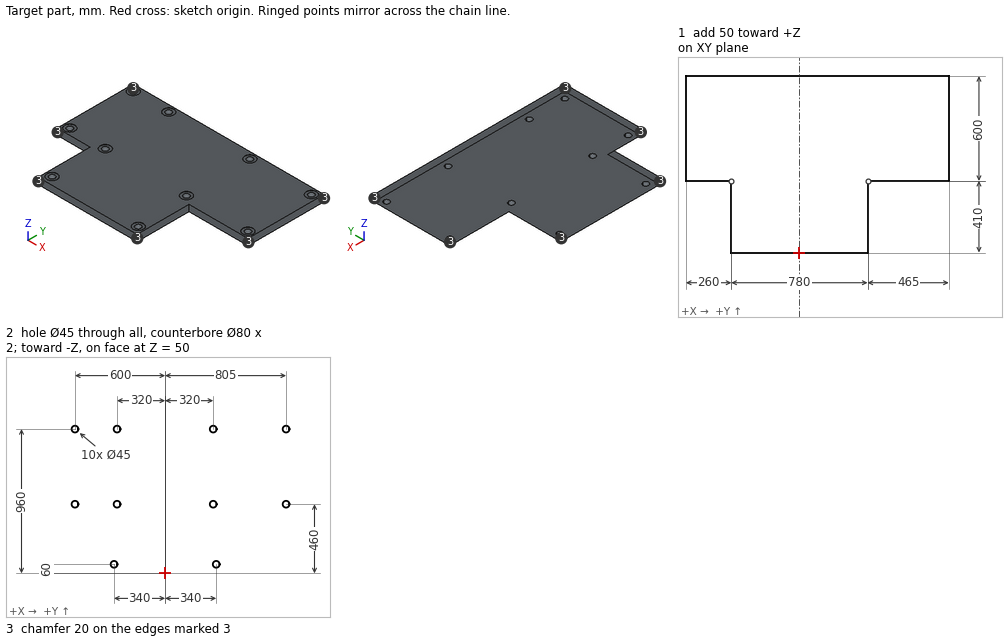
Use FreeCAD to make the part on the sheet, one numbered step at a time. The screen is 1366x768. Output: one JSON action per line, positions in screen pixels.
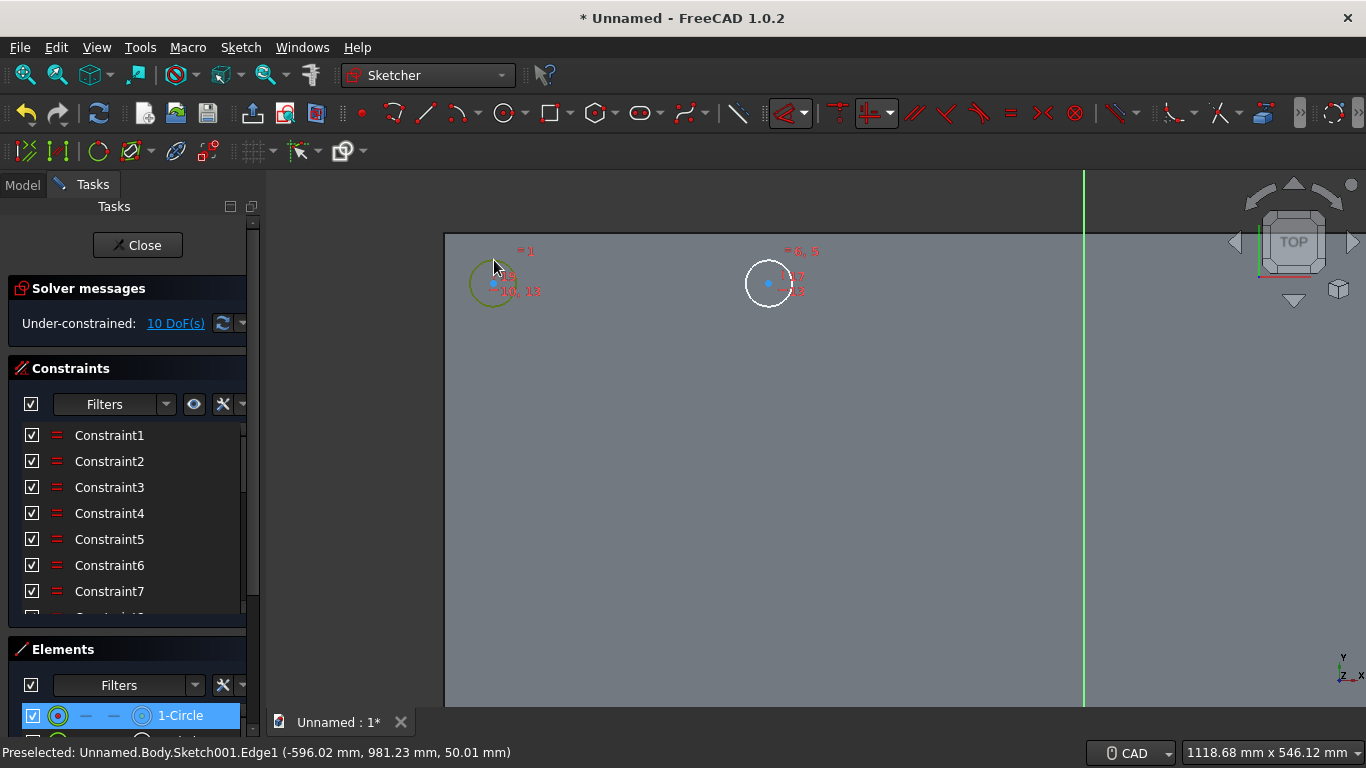
{"action": "key", "text": "k o"}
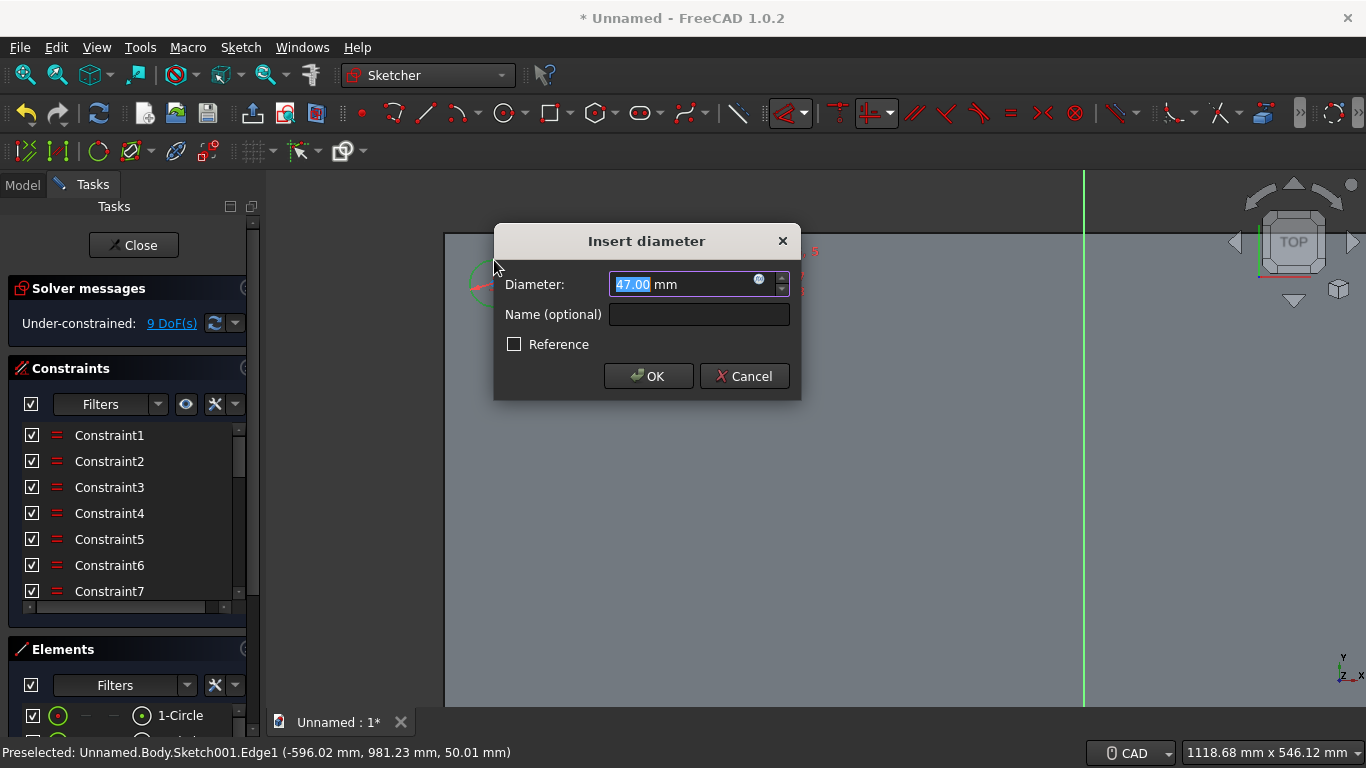
{"action": "type", "text": "45"}
{"action": "key", "text": "Return"}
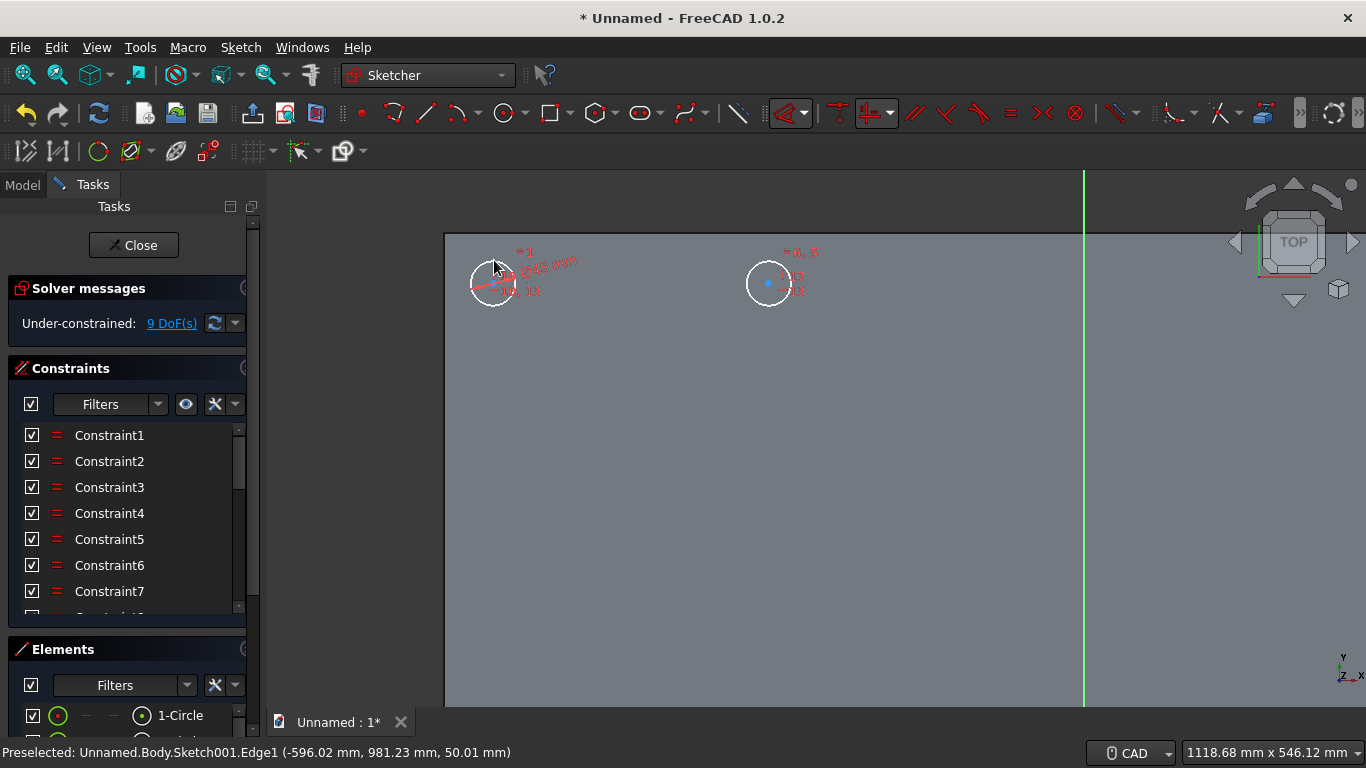
{"action": "scroll", "coordinate": [493, 262], "scroll_direction": "down", "scroll_amount": 5}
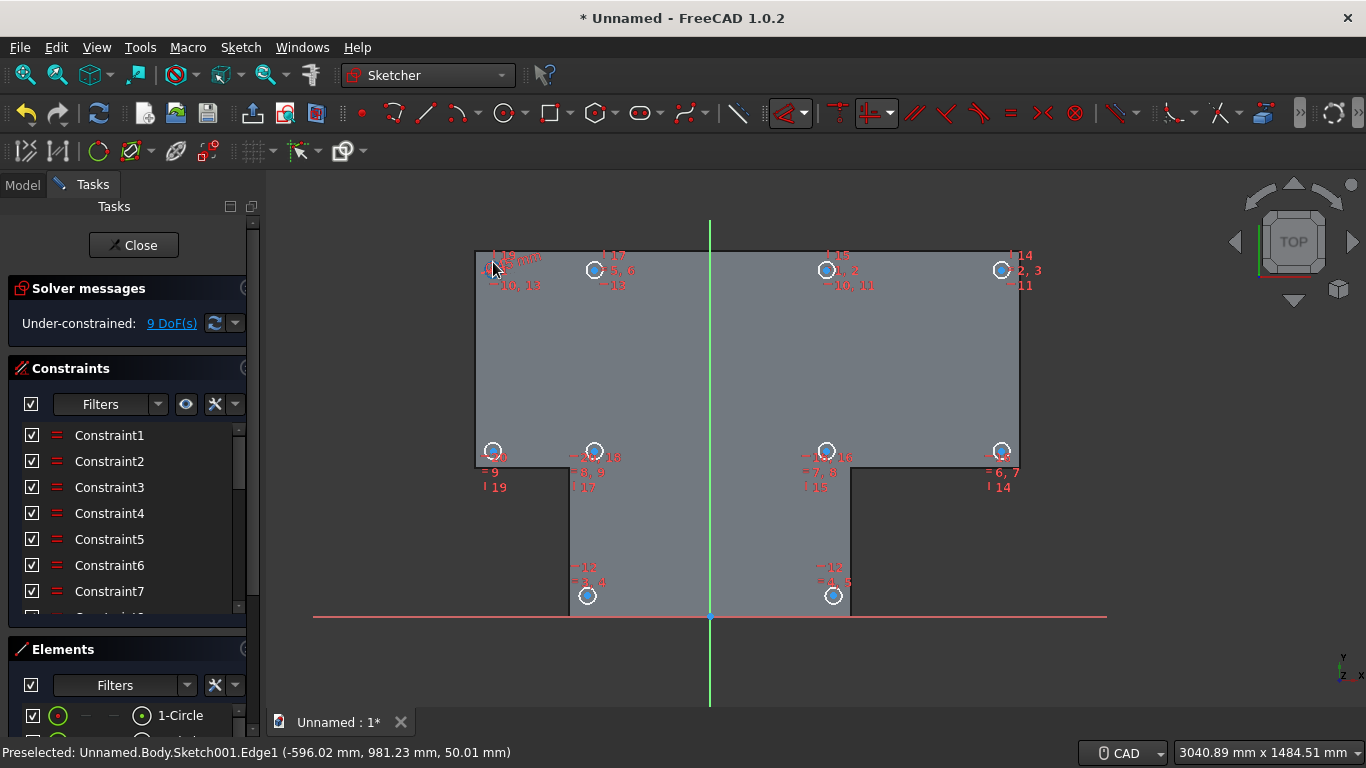
{"action": "scroll", "coordinate": [588, 596], "scroll_direction": "up", "scroll_amount": 4}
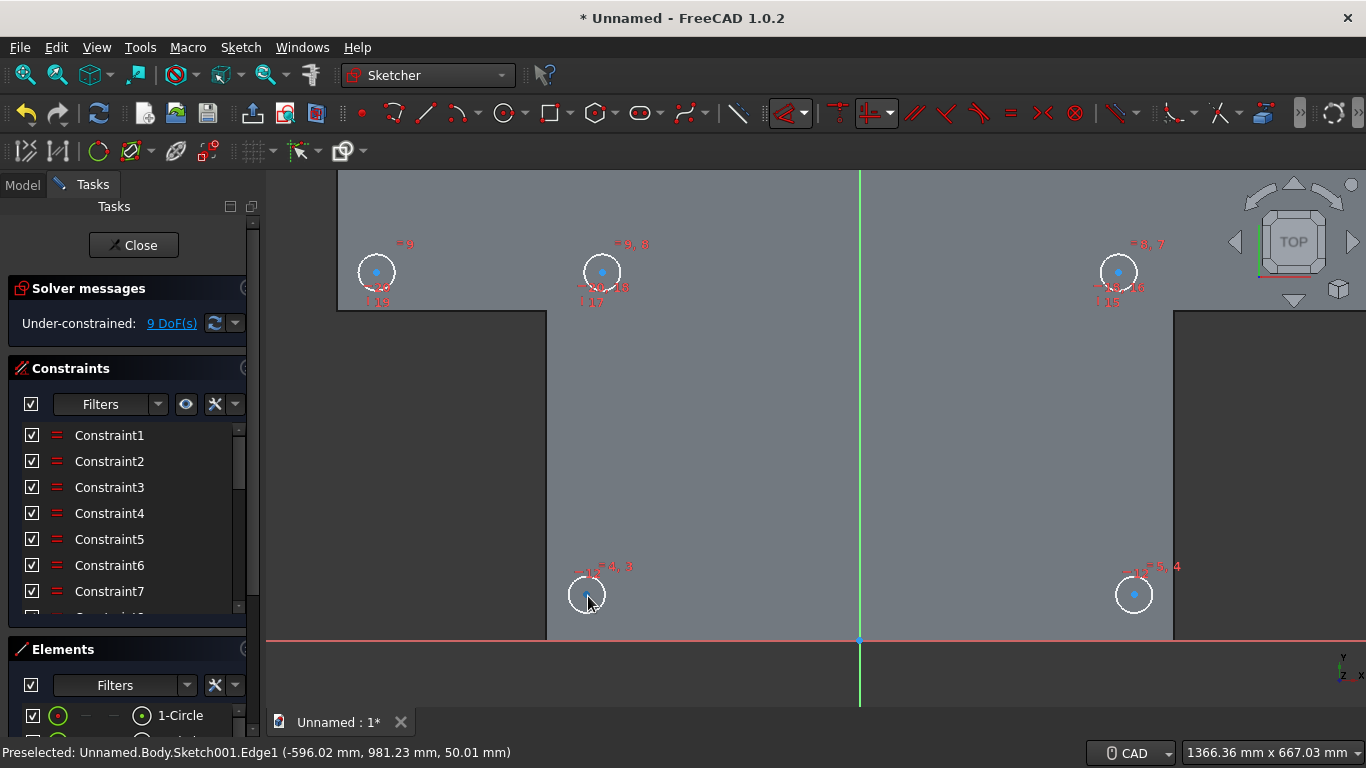
{"action": "left_click", "coordinate": [587, 595]}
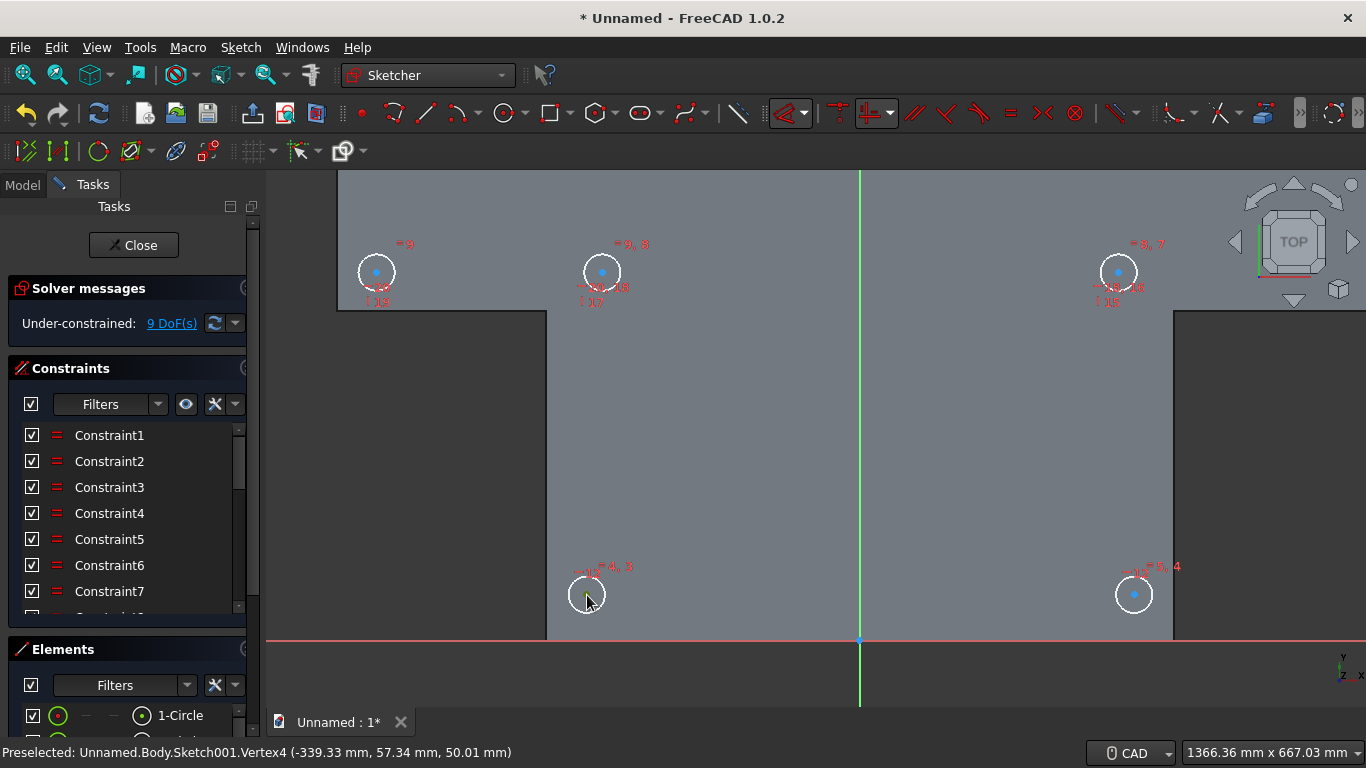
{"action": "left_click", "coordinate": [806, 114]}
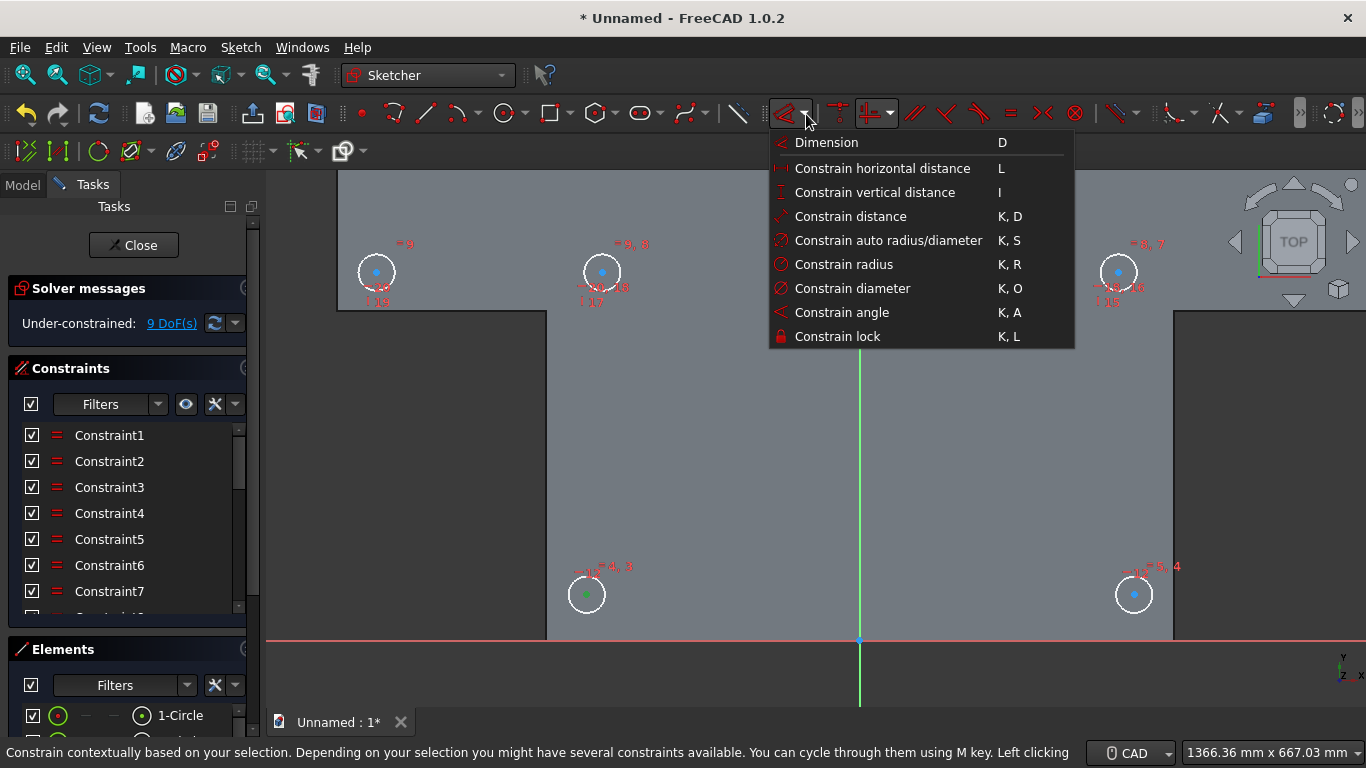
{"action": "left_click", "coordinate": [922, 192]}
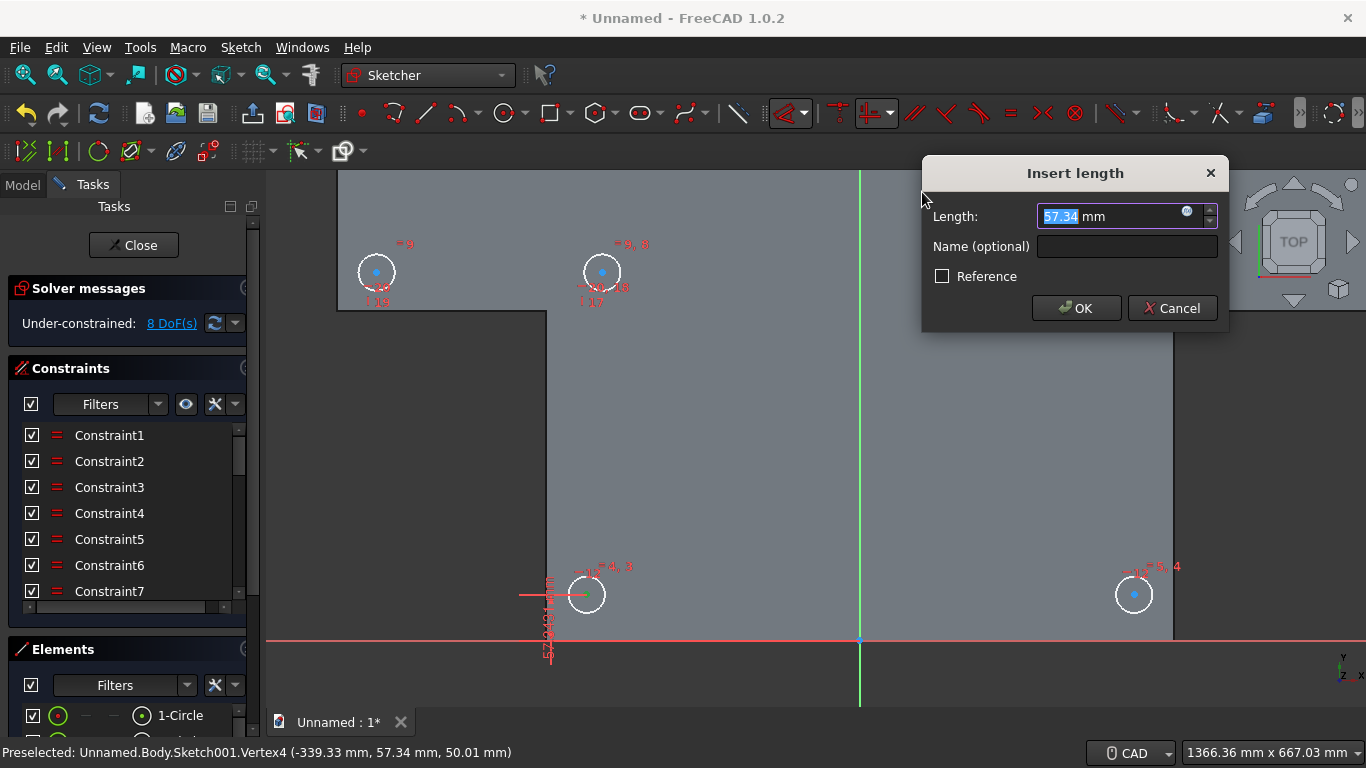
{"action": "type", "text": "60"}
{"action": "key", "text": "Return"}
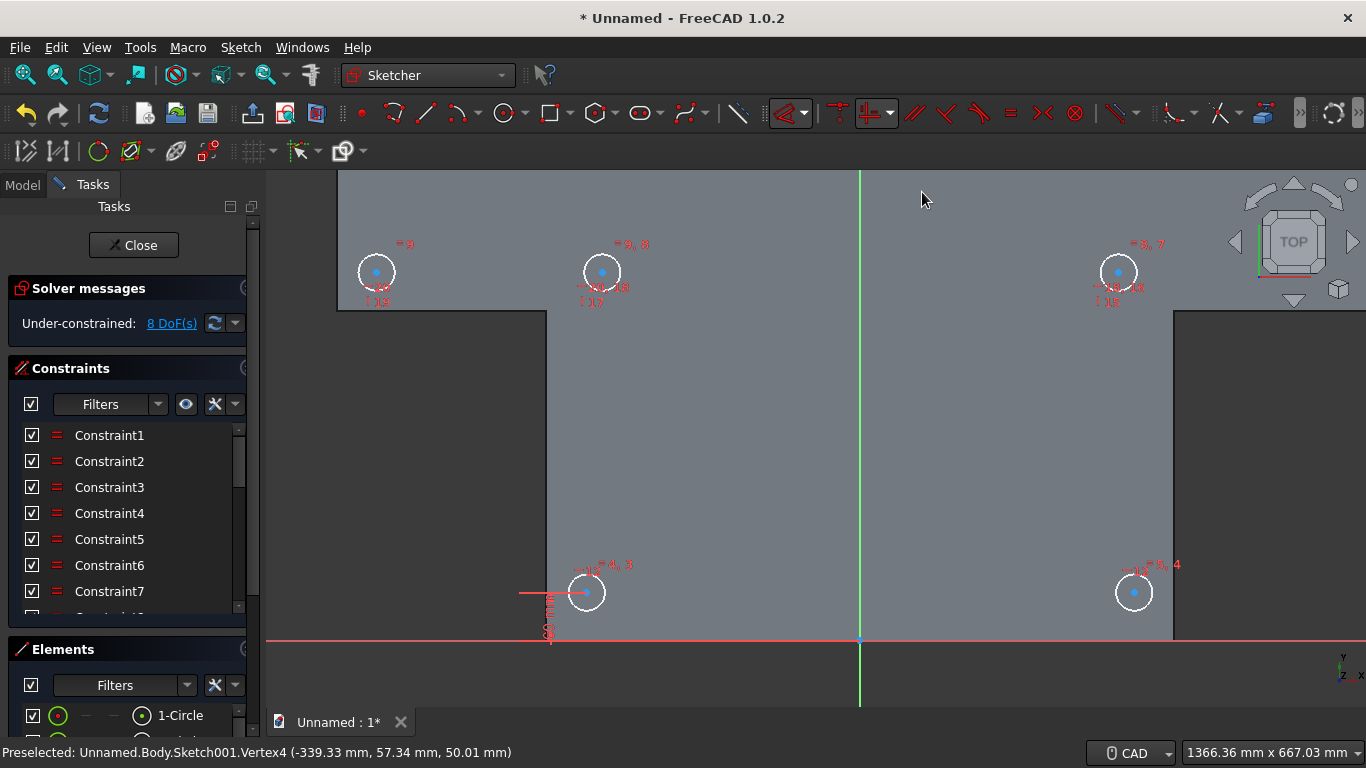
{"action": "scroll", "coordinate": [588, 596], "scroll_direction": "down", "scroll_amount": 4}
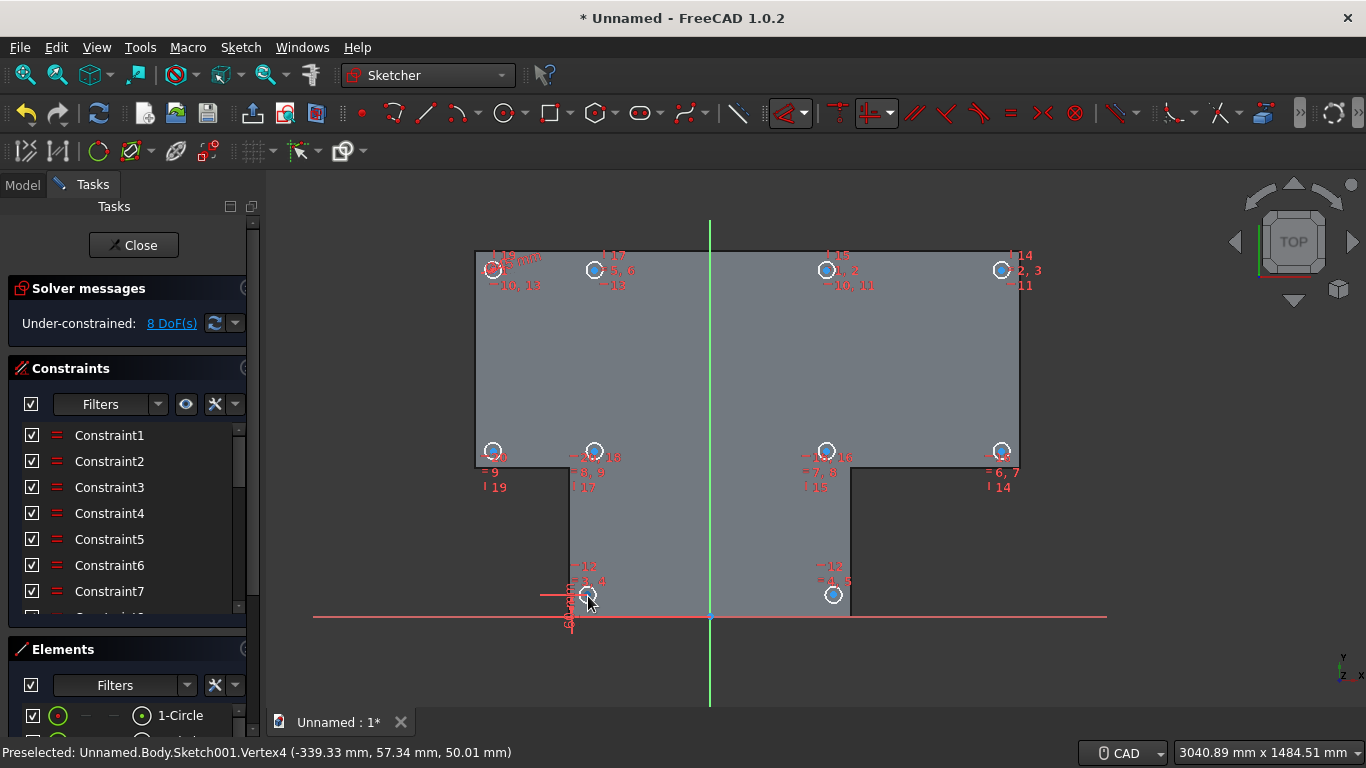
{"action": "left_click", "coordinate": [493, 270]}